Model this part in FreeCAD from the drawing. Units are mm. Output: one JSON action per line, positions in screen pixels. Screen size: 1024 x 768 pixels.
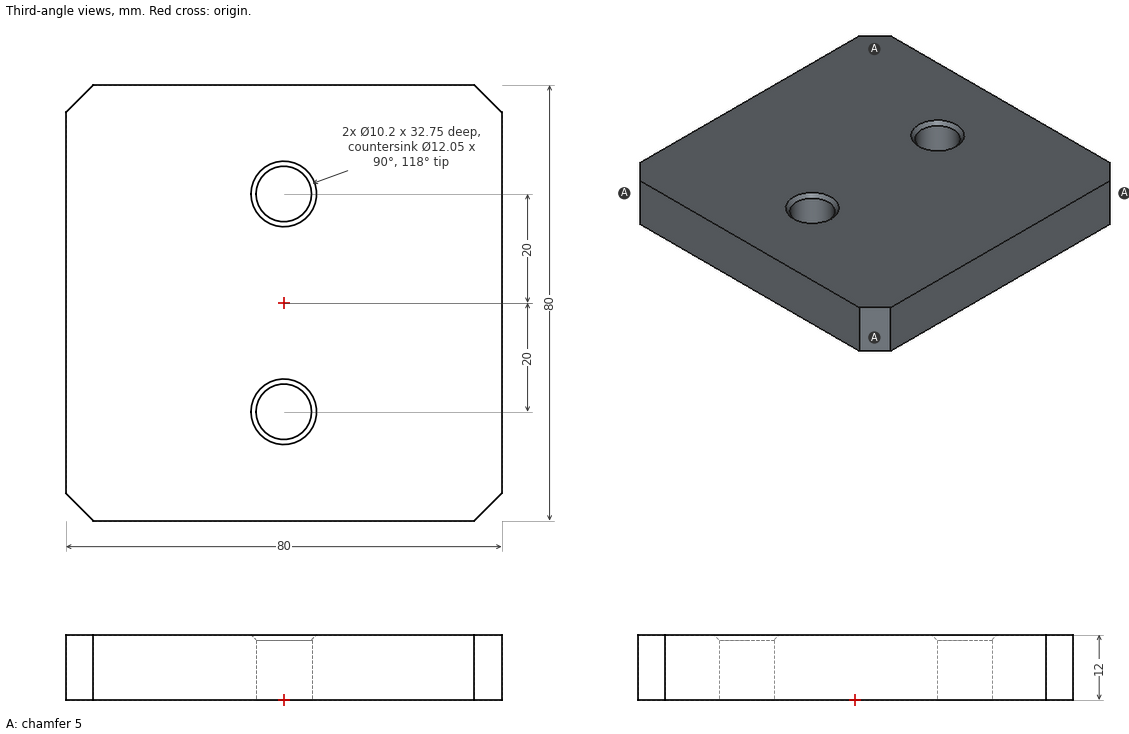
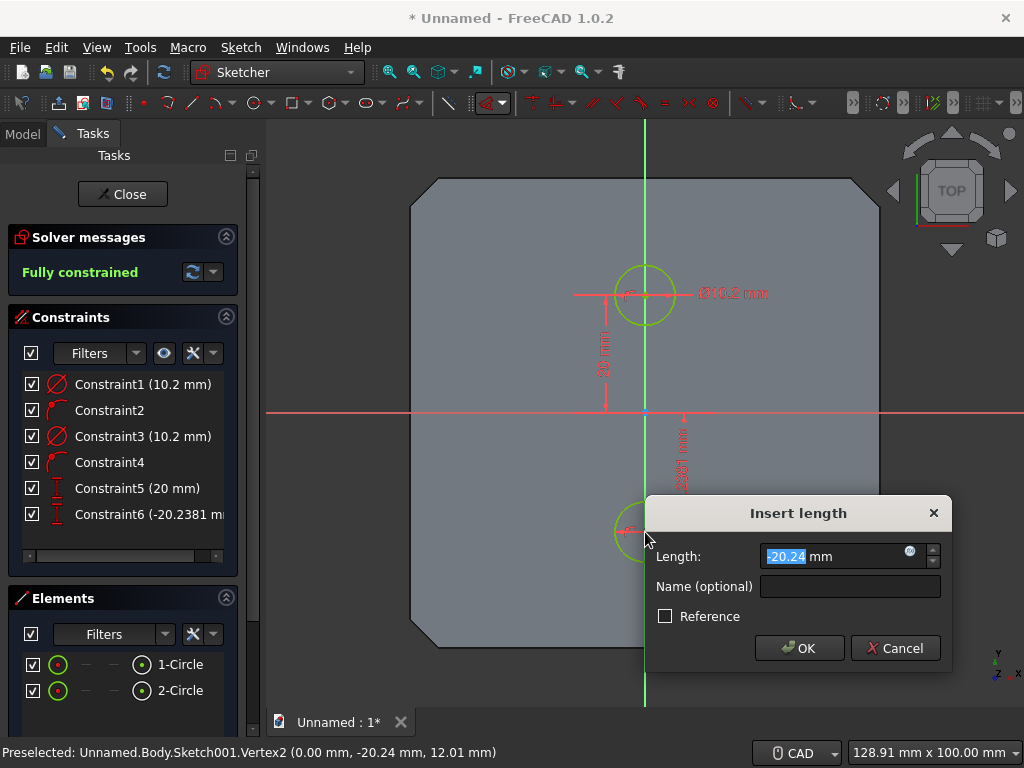
{"action": "type", "text": "-20"}
{"action": "key", "text": "Return"}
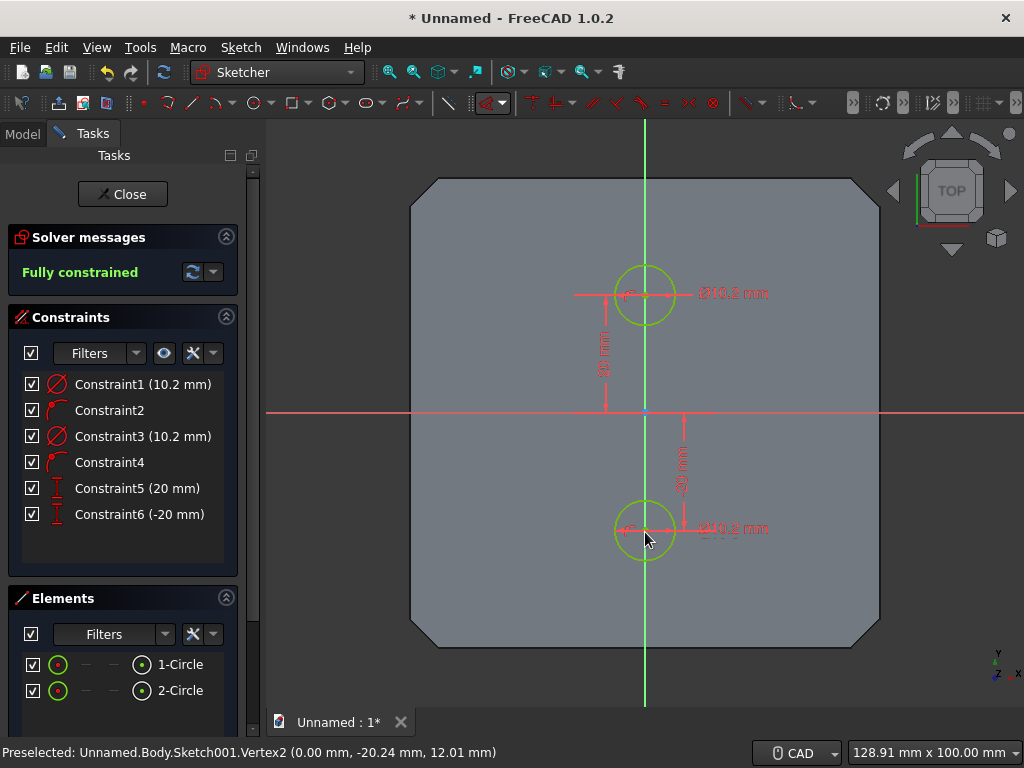
{"action": "left_click", "coordinate": [123, 194]}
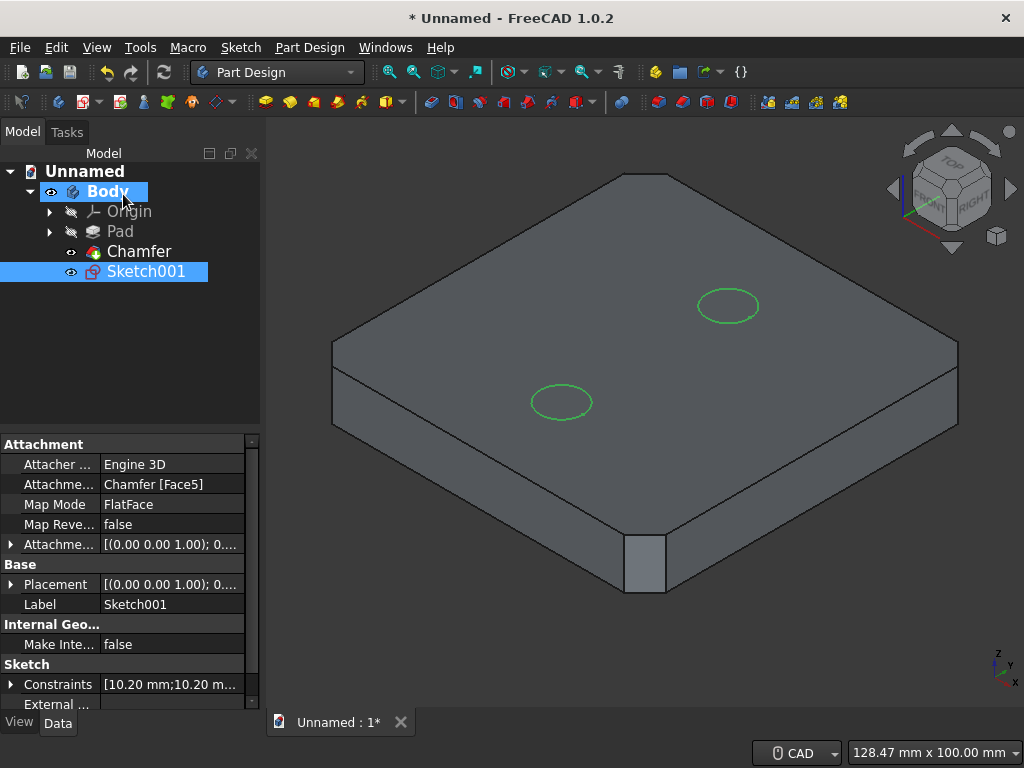
{"action": "left_click", "coordinate": [456, 102]}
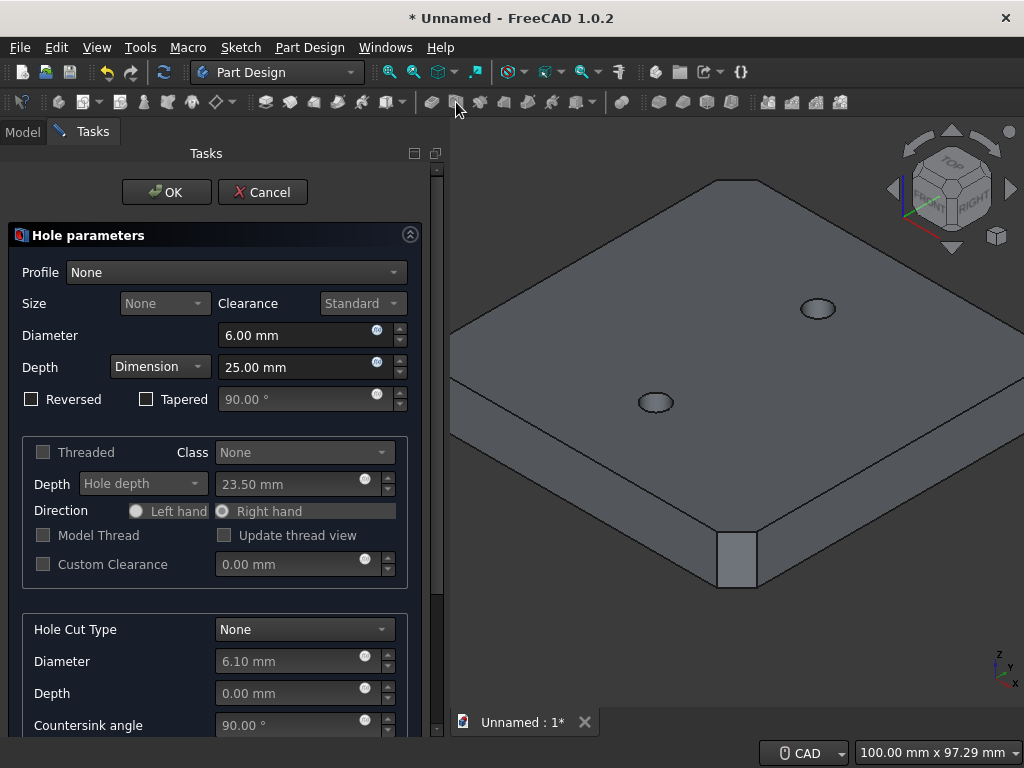
{"action": "triple_click", "coordinate": [305, 335]}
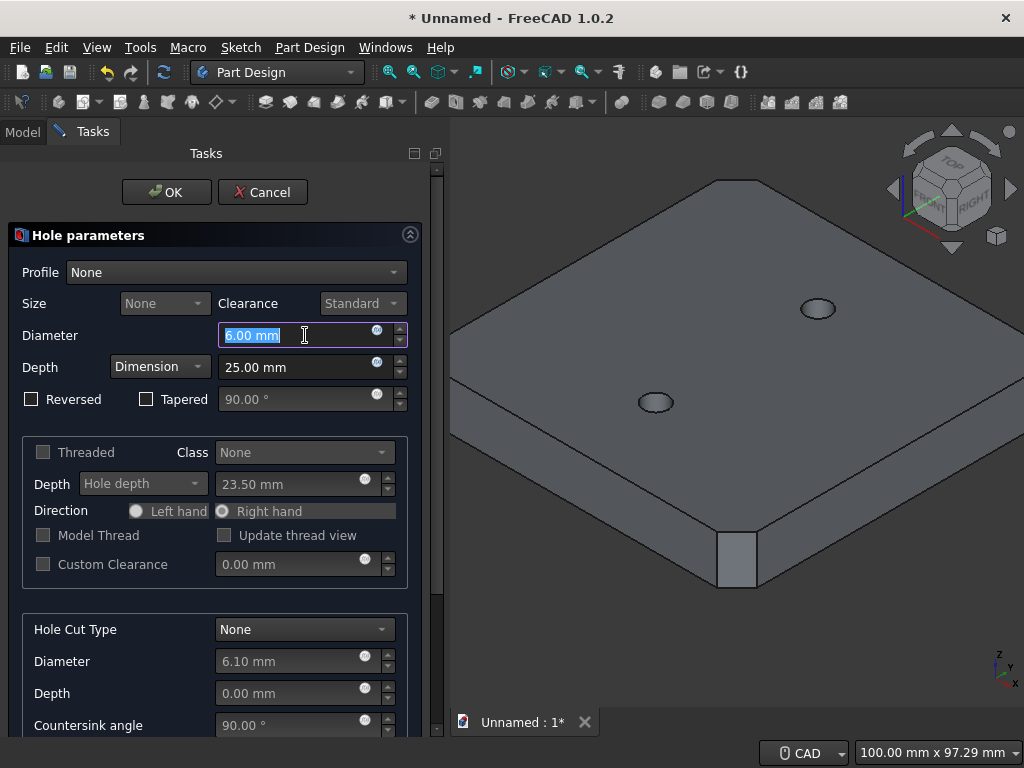
{"action": "type", "text": "10.2"}
{"action": "key", "text": "Tab"}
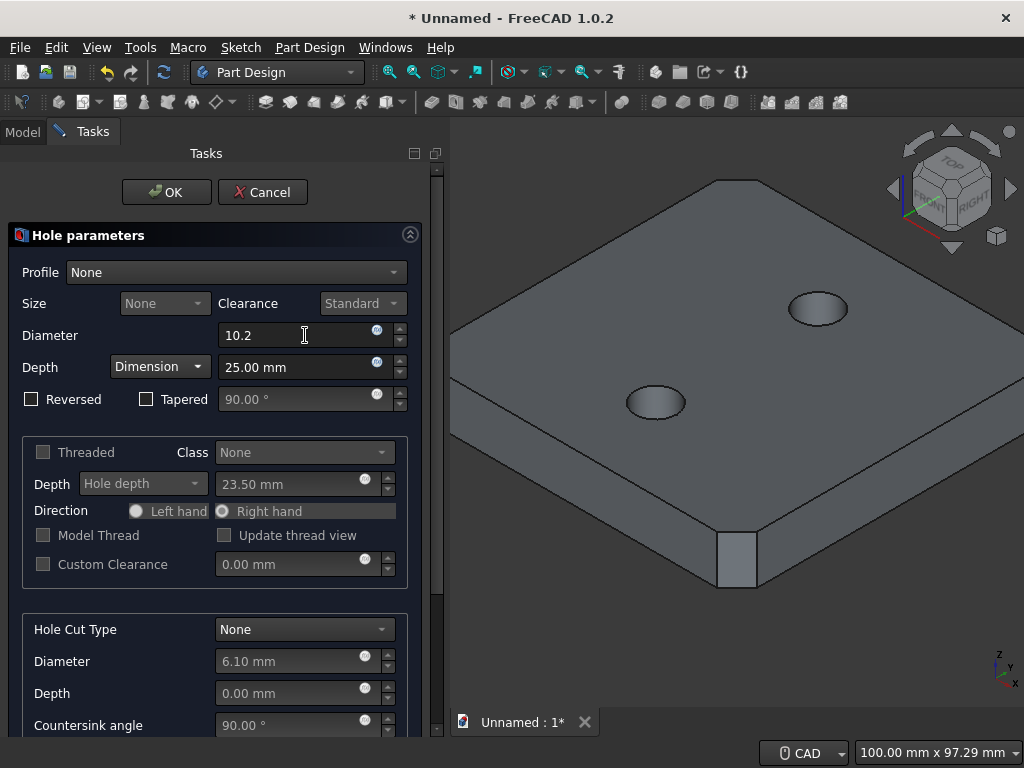
{"action": "triple_click", "coordinate": [305, 367]}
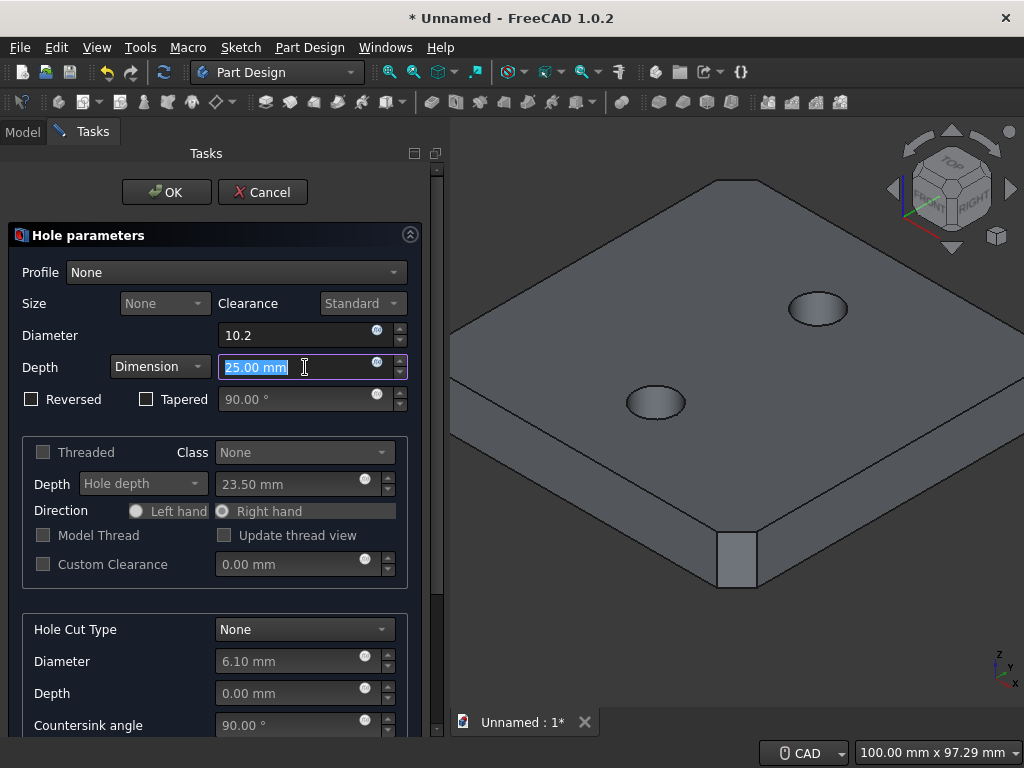
{"action": "type", "text": "32.75"}
{"action": "key", "text": "Tab"}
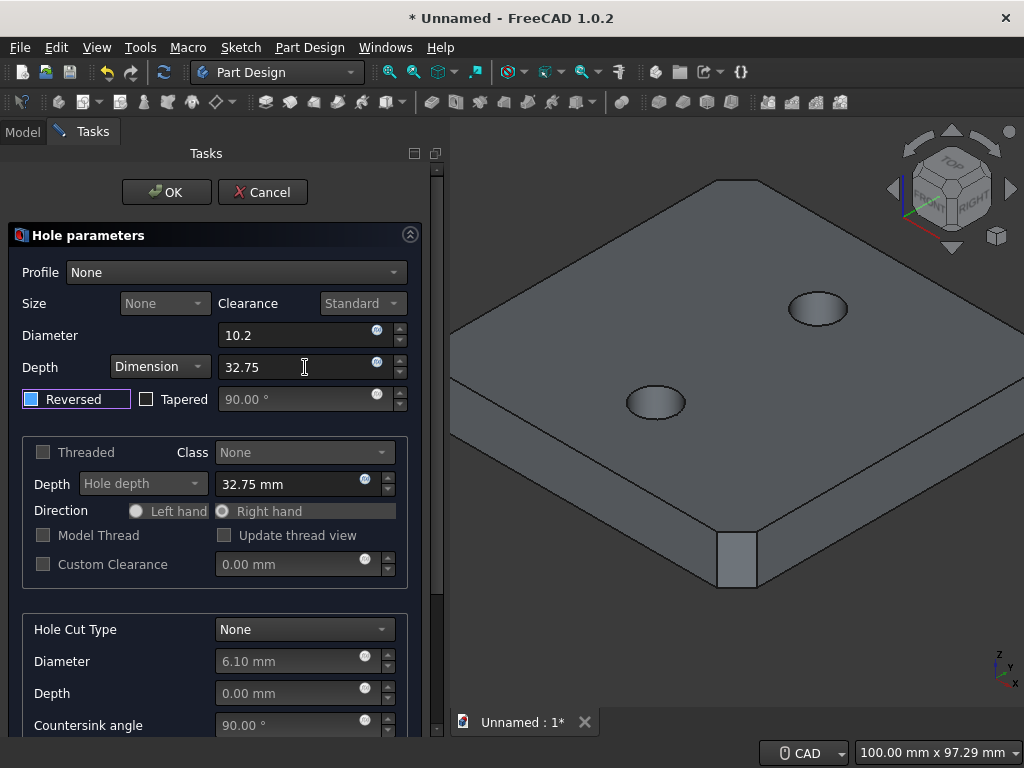
{"action": "left_click", "coordinate": [306, 630]}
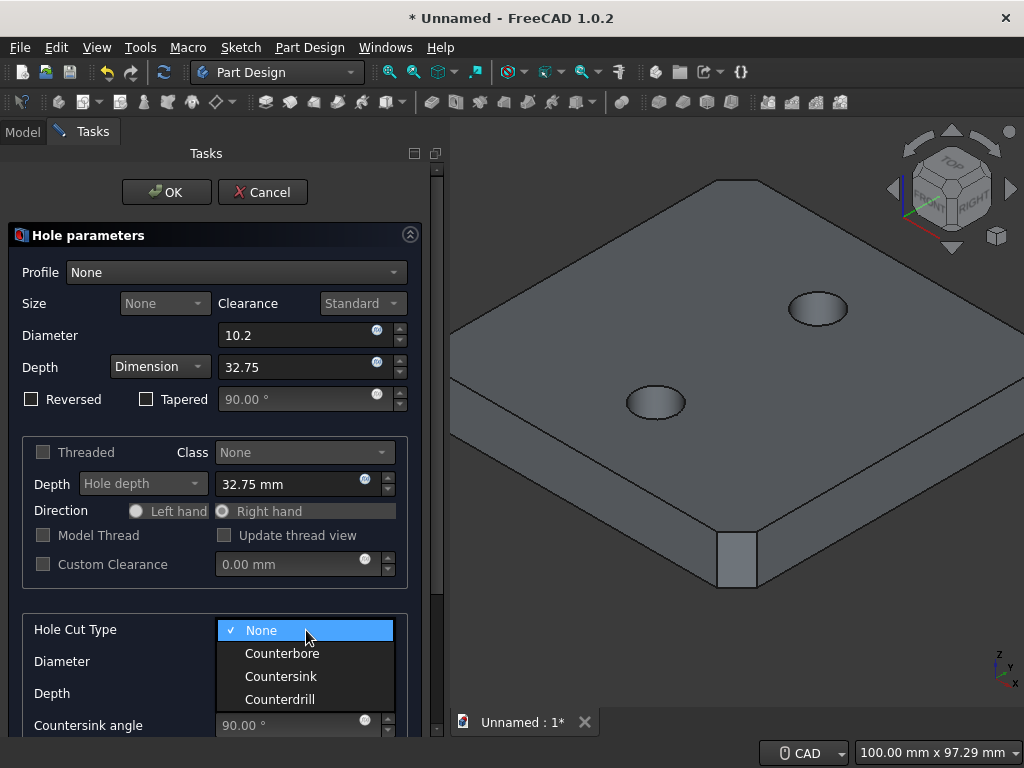
{"action": "left_click", "coordinate": [304, 676]}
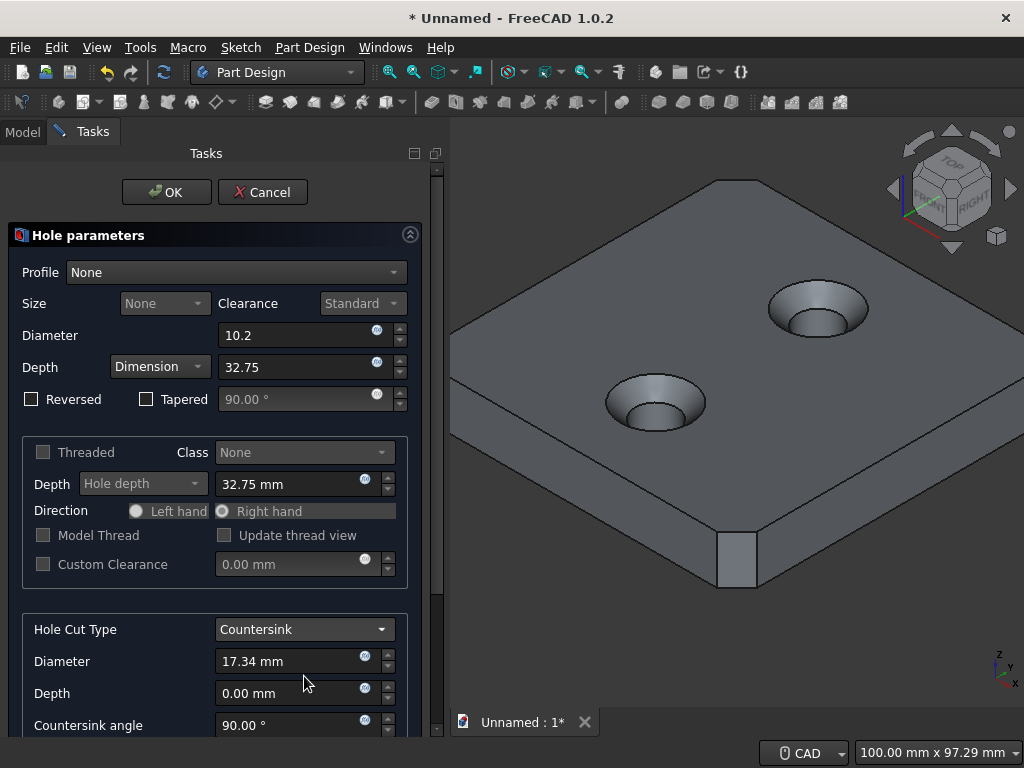
{"action": "triple_click", "coordinate": [298, 661]}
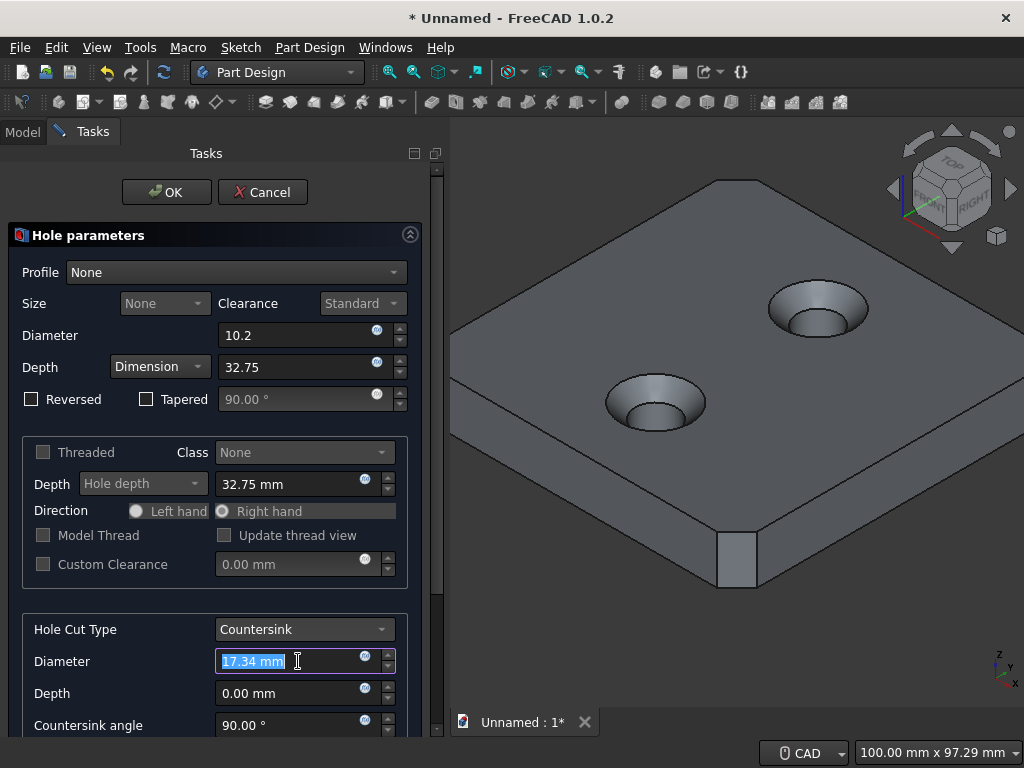
{"action": "type", "text": "12.05"}
{"action": "key", "text": "Tab"}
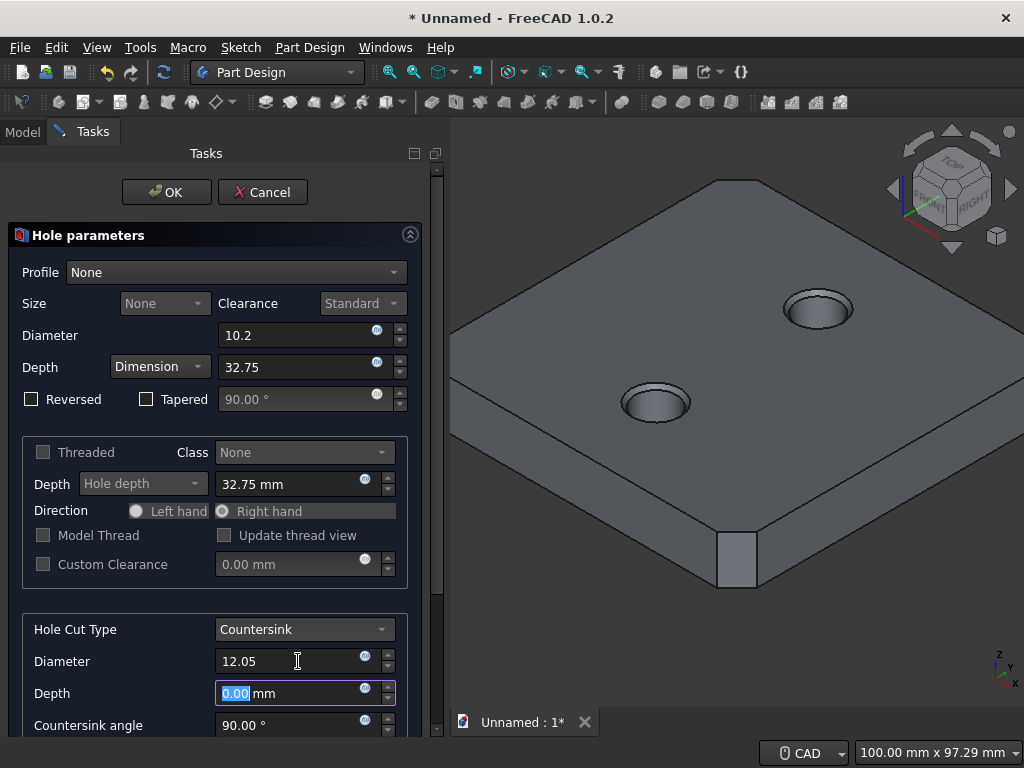
{"action": "left_click", "coordinate": [167, 192]}